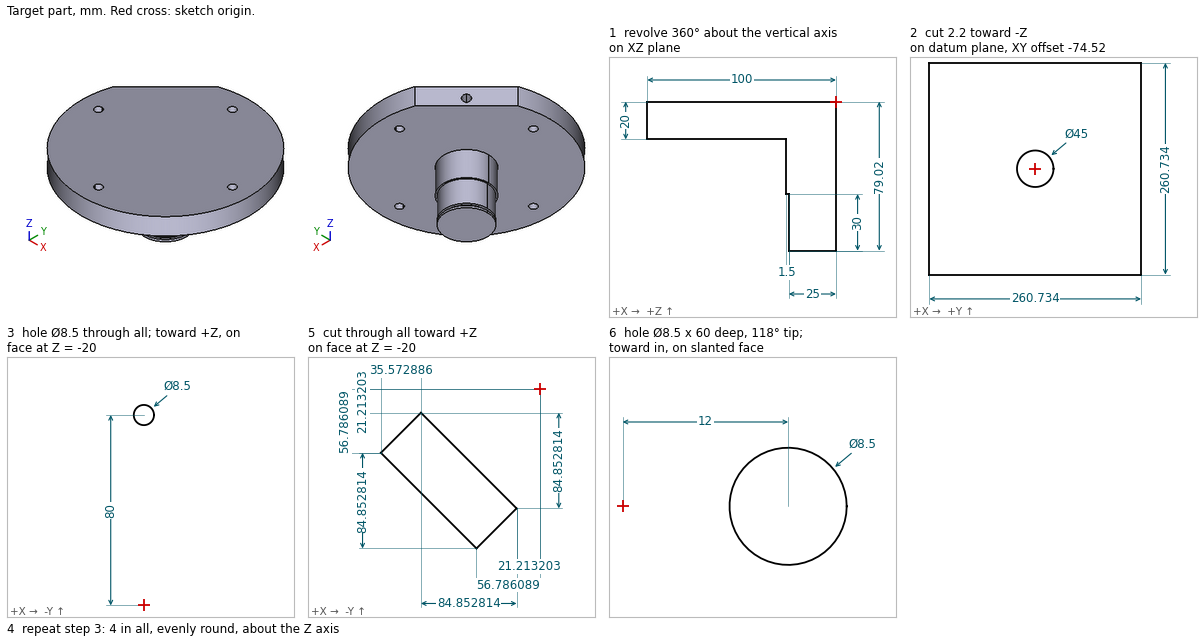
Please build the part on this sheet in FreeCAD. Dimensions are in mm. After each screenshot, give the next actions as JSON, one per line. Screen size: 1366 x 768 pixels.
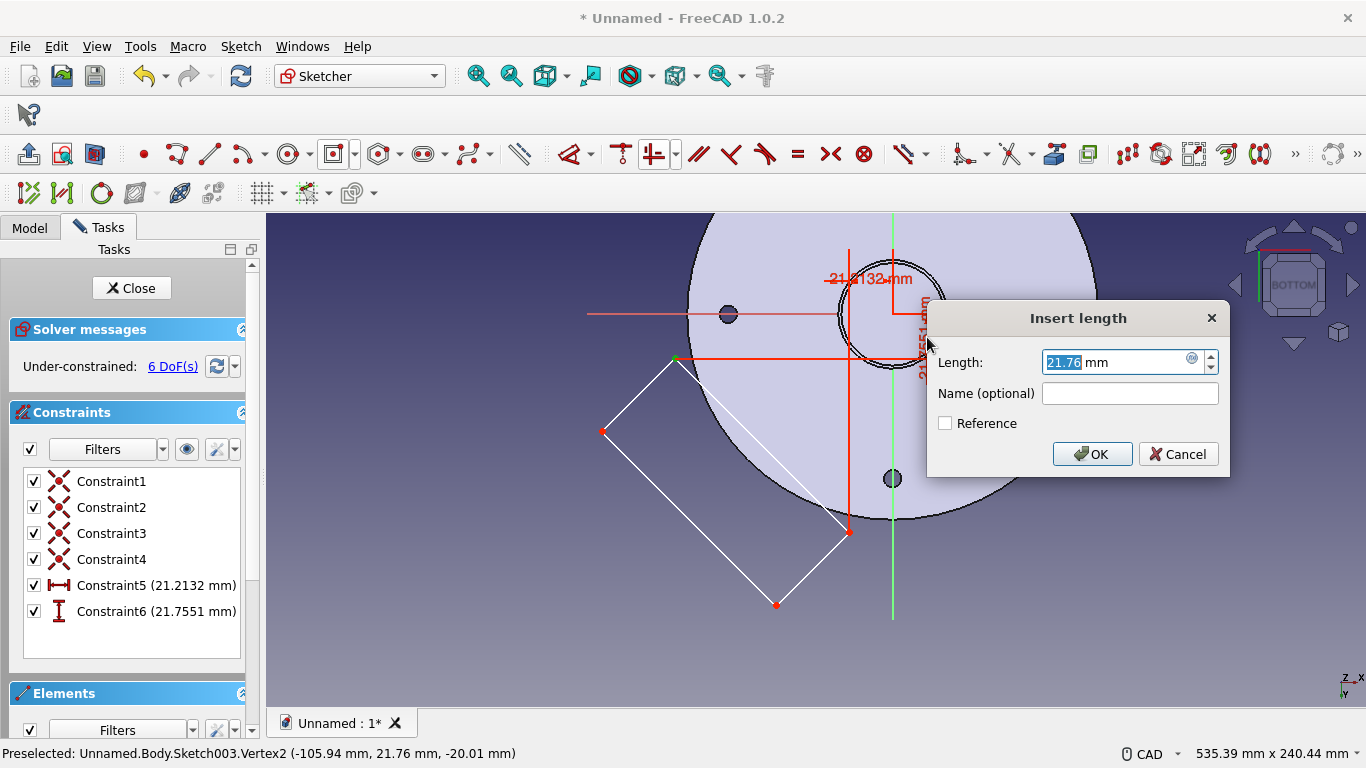
{"action": "type", "text": "21.213203"}
{"action": "key", "text": "Return"}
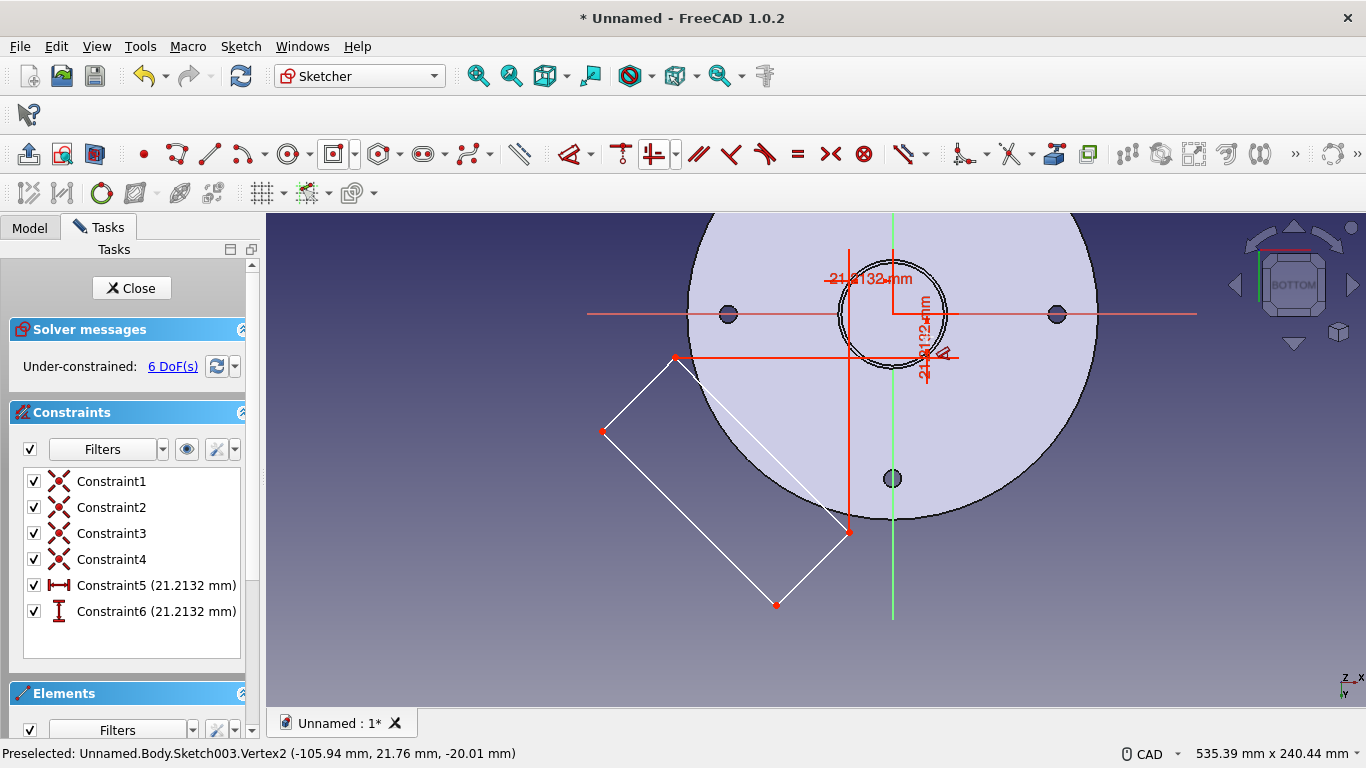
{"action": "left_click", "coordinate": [602, 432]}
{"action": "left_click", "coordinate": [927, 373]}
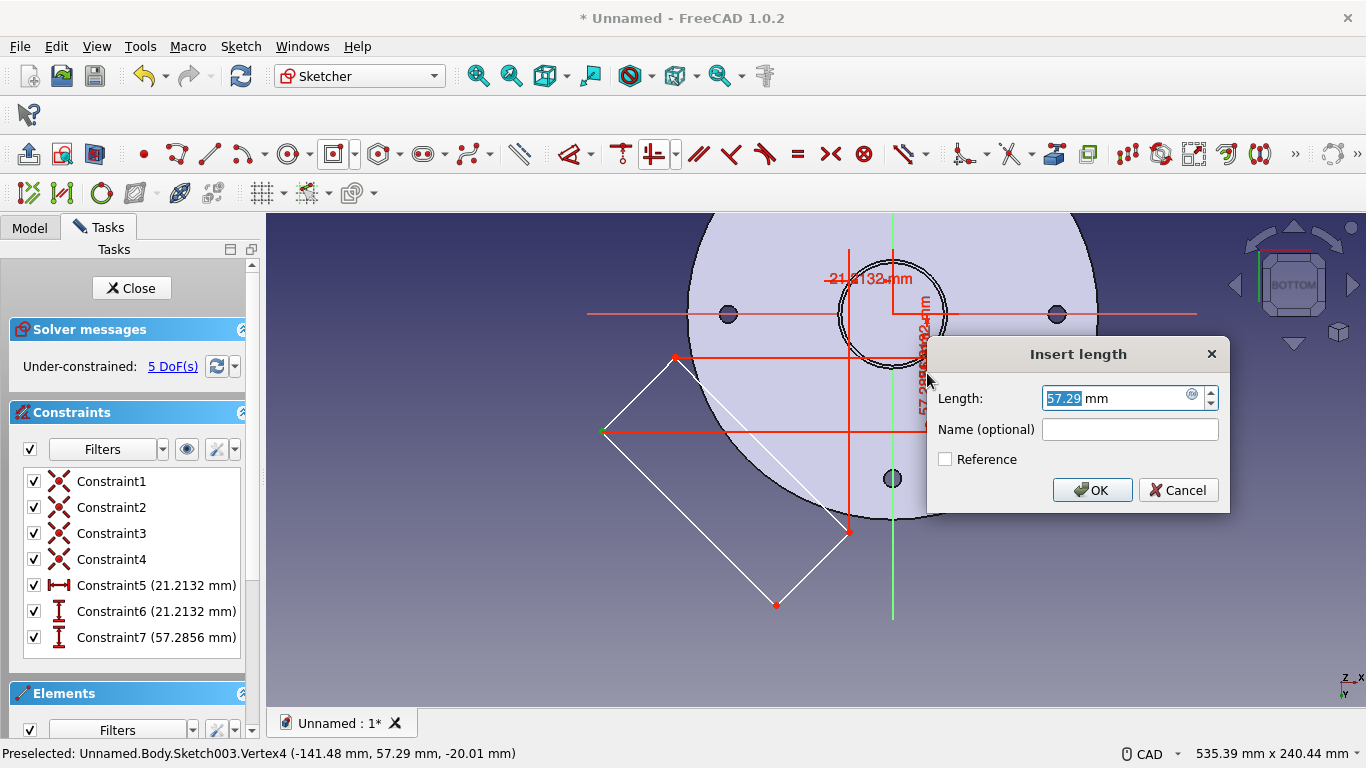
{"action": "type", "text": "56.786089"}
{"action": "key", "text": "Return"}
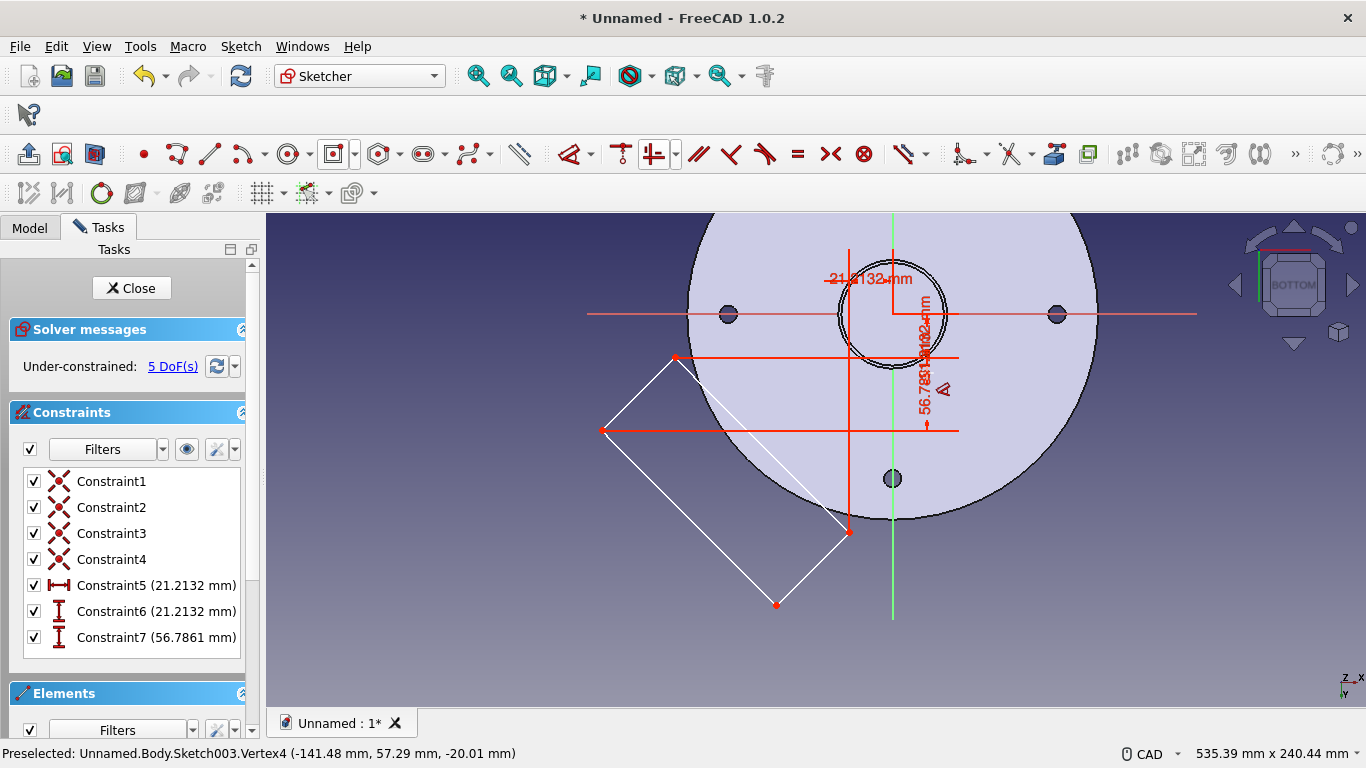
{"action": "left_click", "coordinate": [776, 606]}
{"action": "left_click", "coordinate": [834, 640]}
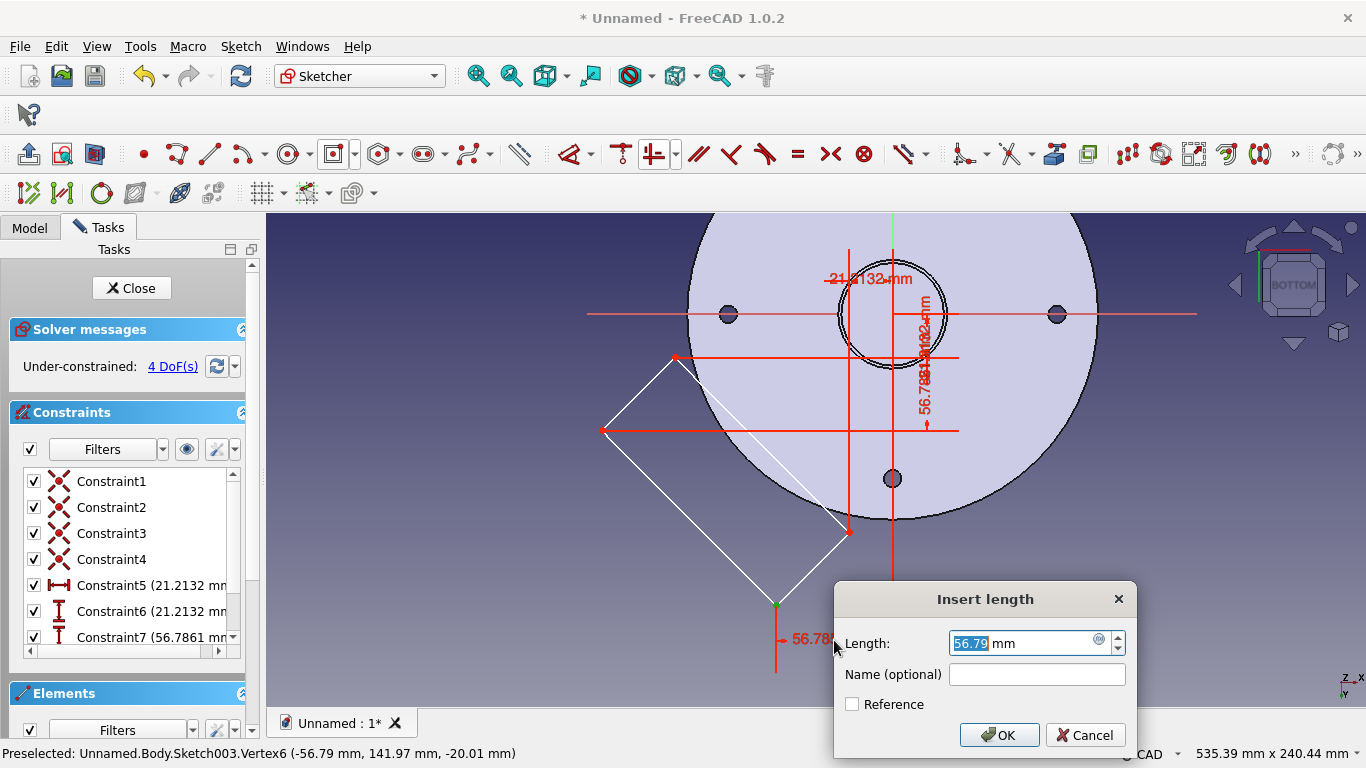
{"action": "type", "text": "56.786089"}
{"action": "key", "text": "Return"}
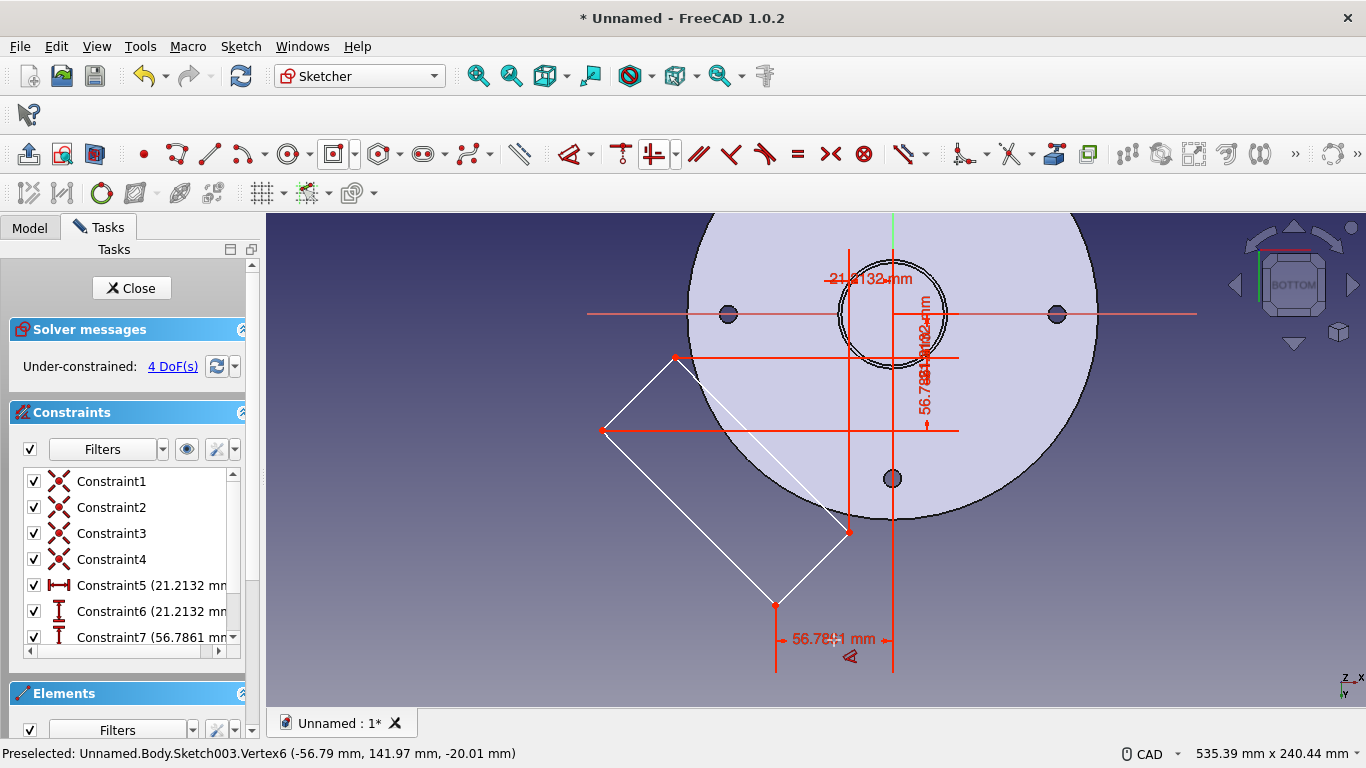
{"action": "left_click", "coordinate": [797, 480]}
{"action": "left_click", "coordinate": [762, 567]}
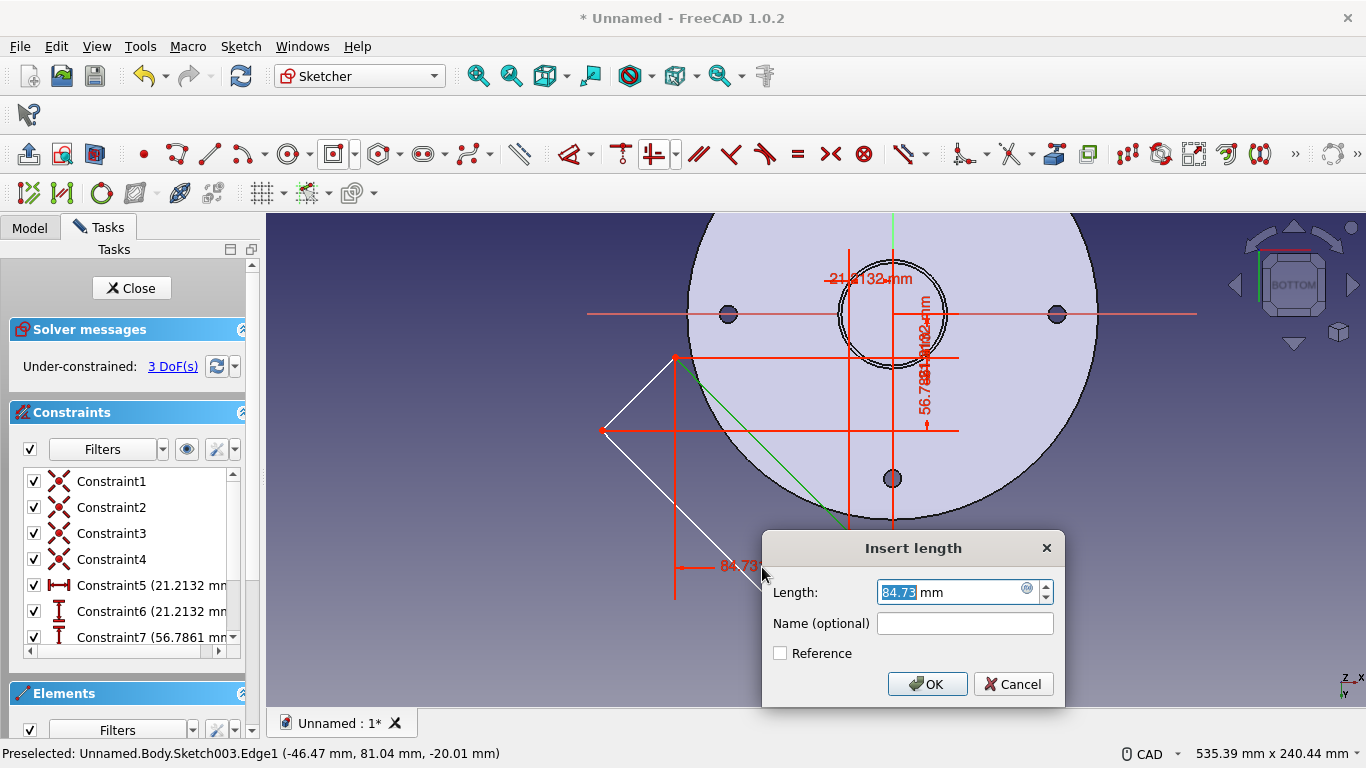
{"action": "type", "text": "84.852814"}
{"action": "key", "text": "Return"}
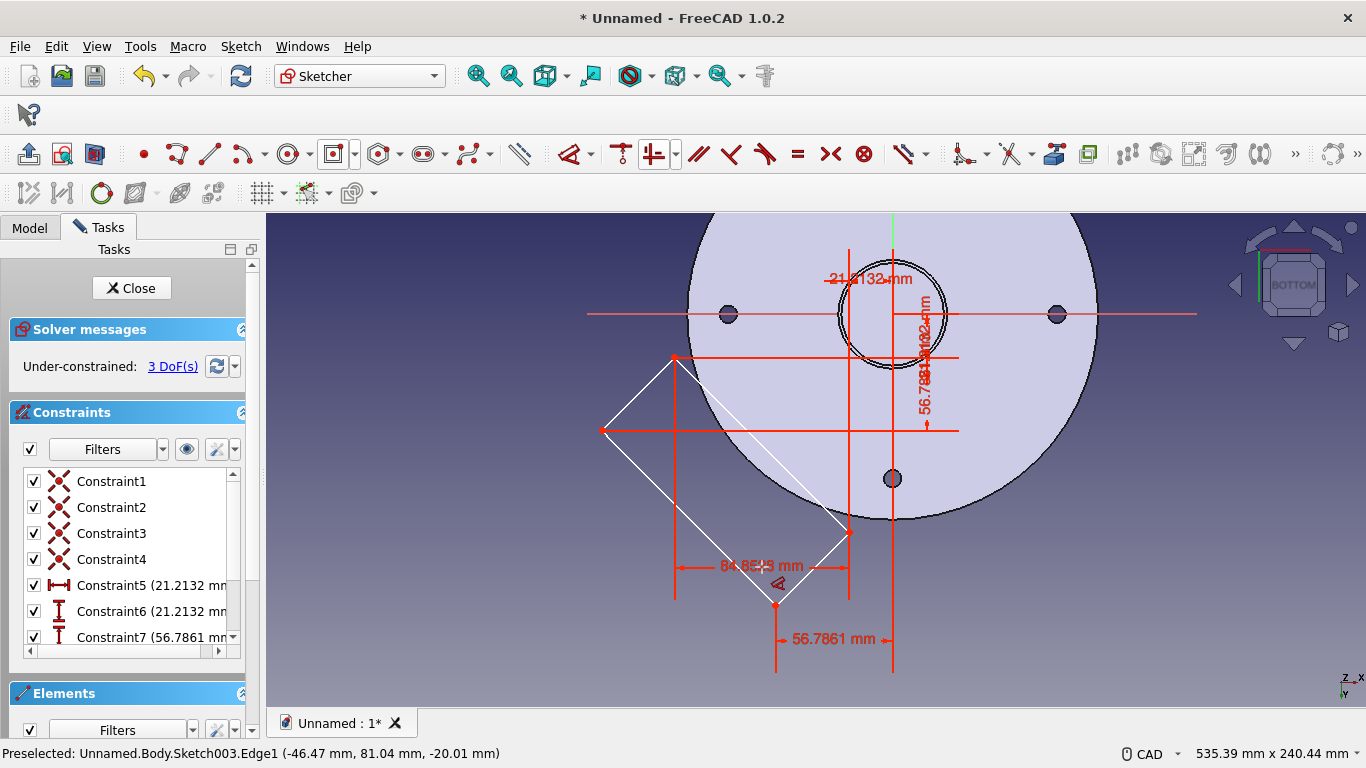
{"action": "left_click", "coordinate": [797, 480]}
{"action": "left_click", "coordinate": [641, 445]}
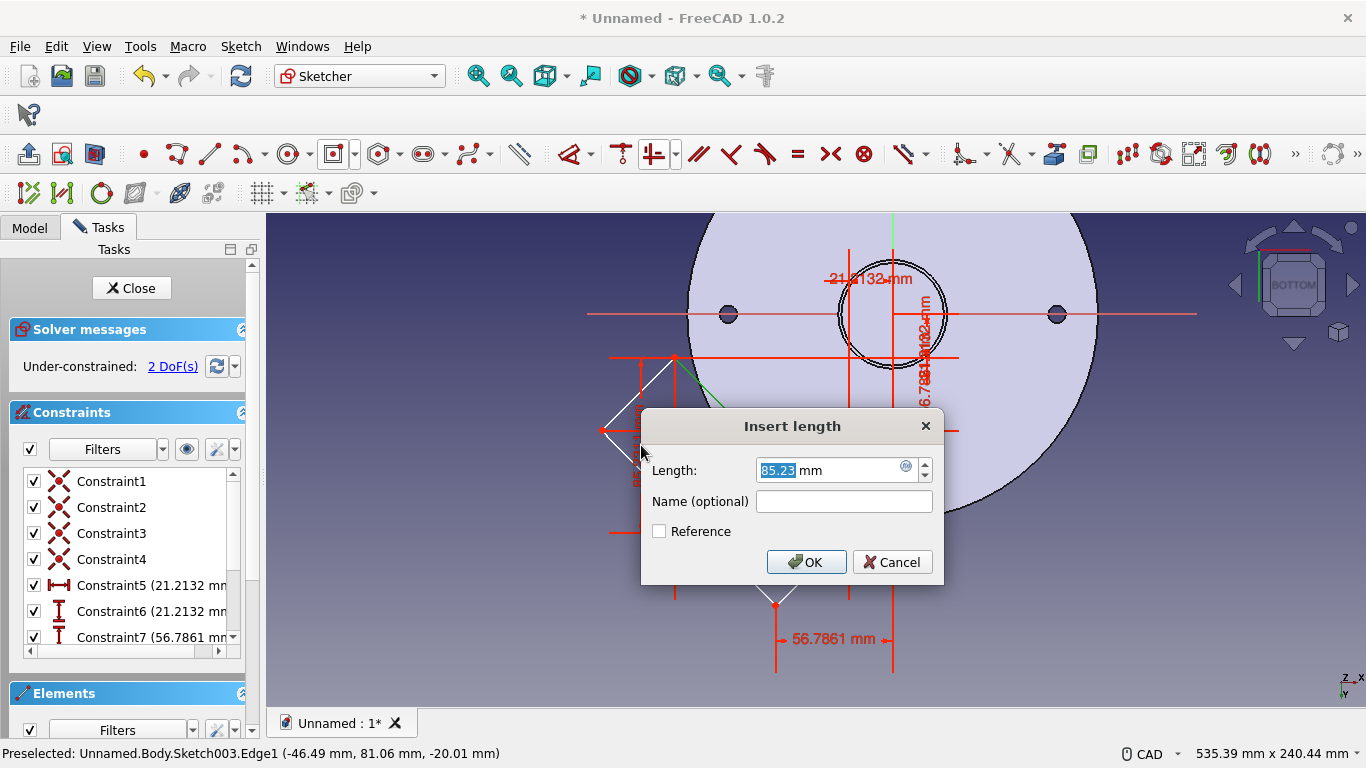
{"action": "type", "text": "84.852814"}
{"action": "key", "text": "Return"}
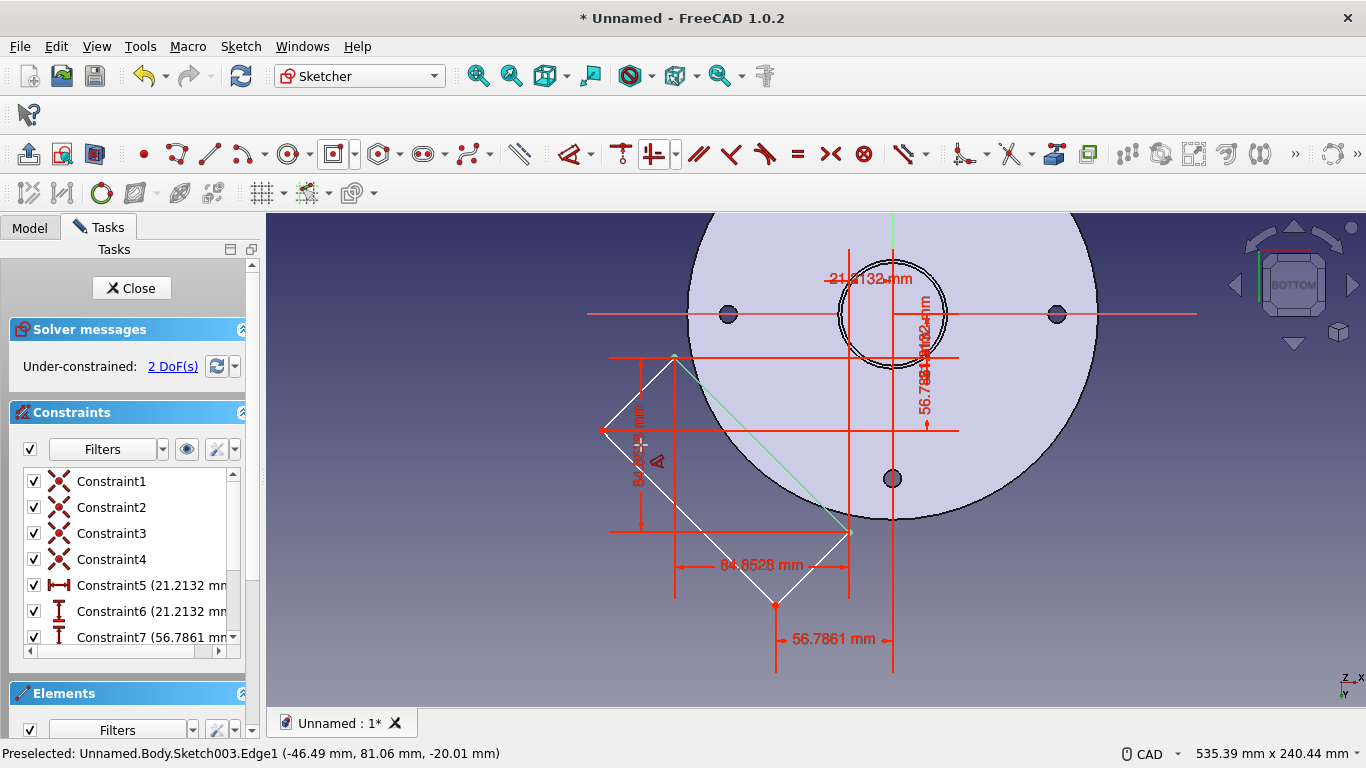
{"action": "left_click", "coordinate": [653, 380]}
{"action": "left_click", "coordinate": [638, 300]}